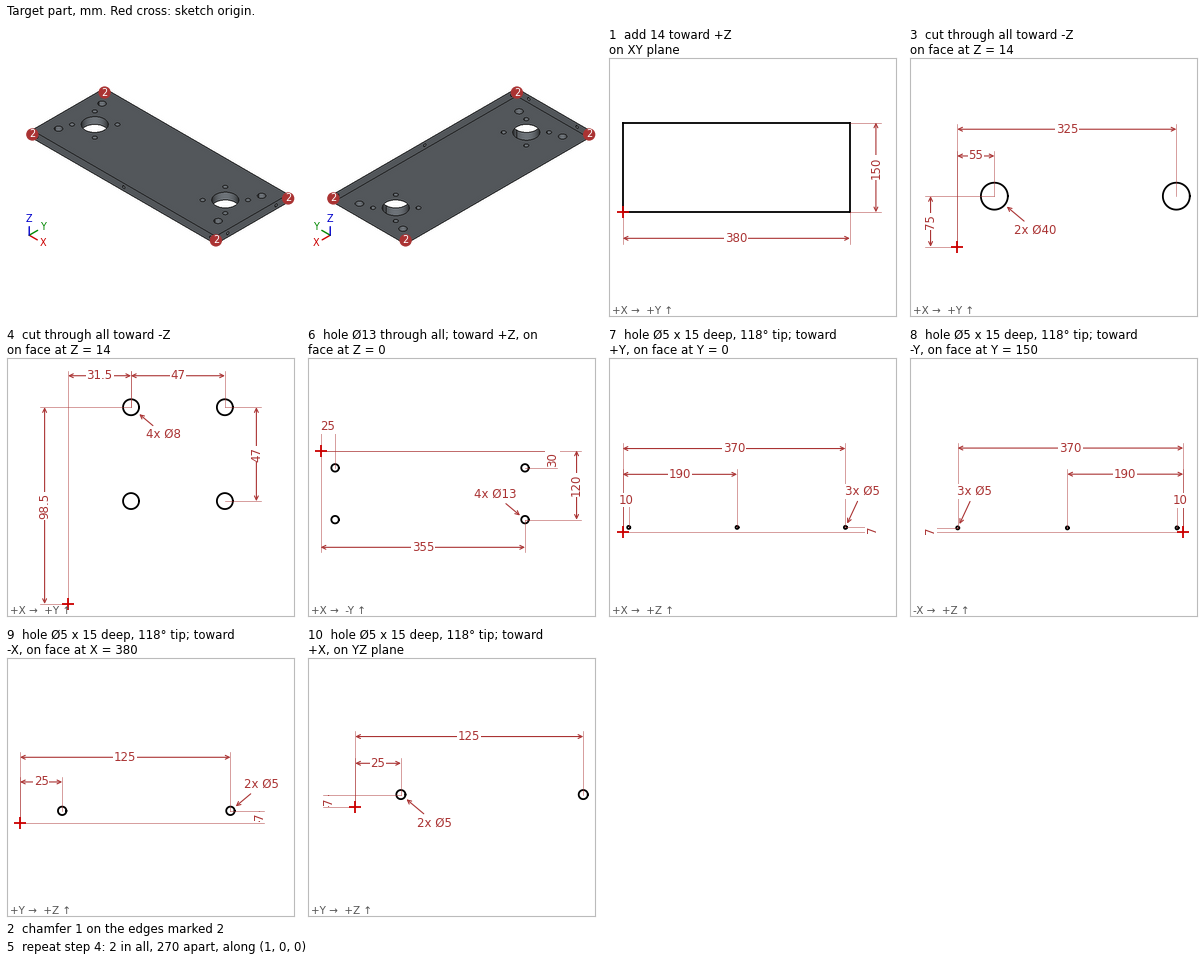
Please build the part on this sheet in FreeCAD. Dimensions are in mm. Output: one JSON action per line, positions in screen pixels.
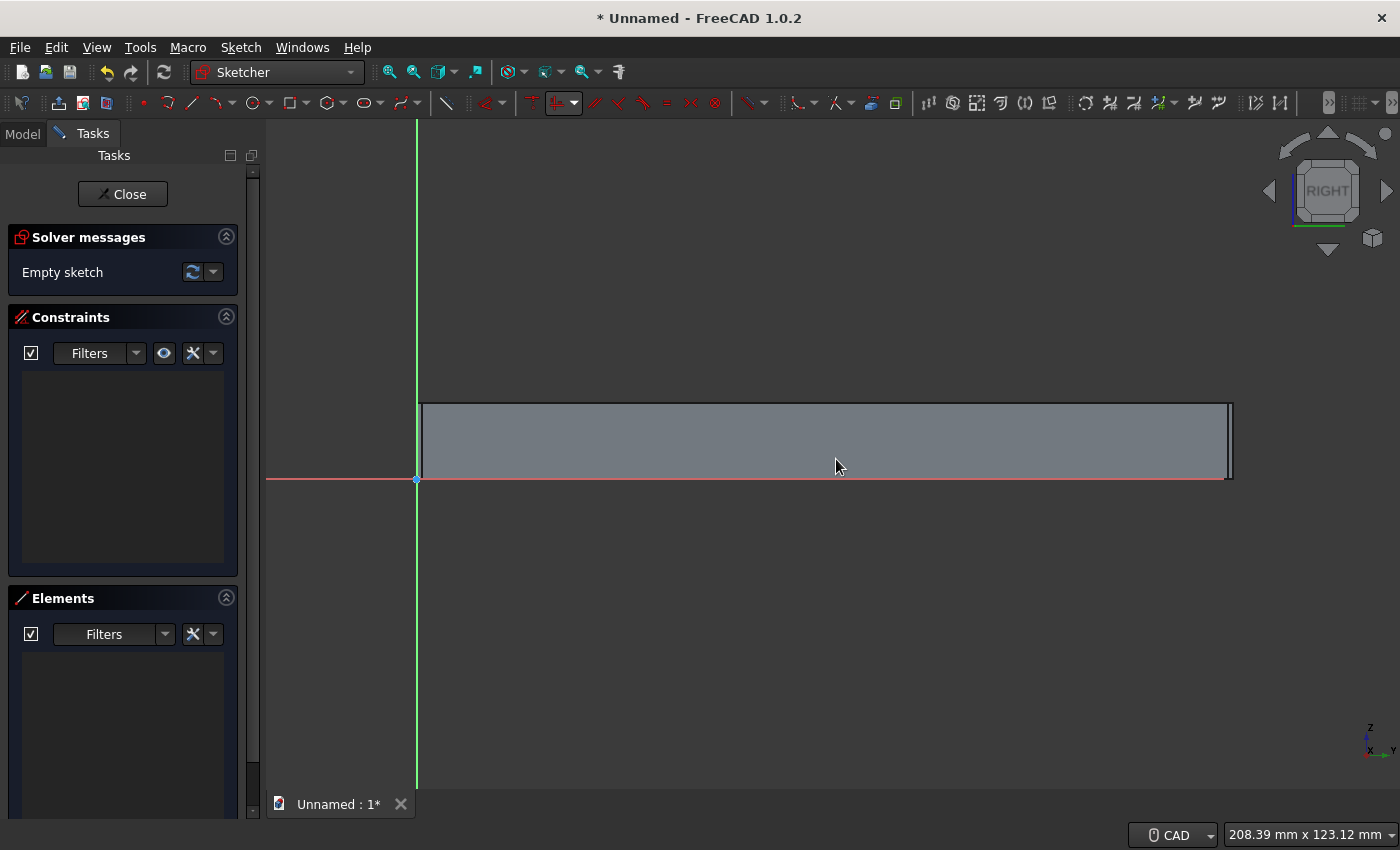
{"action": "key", "text": "g c"}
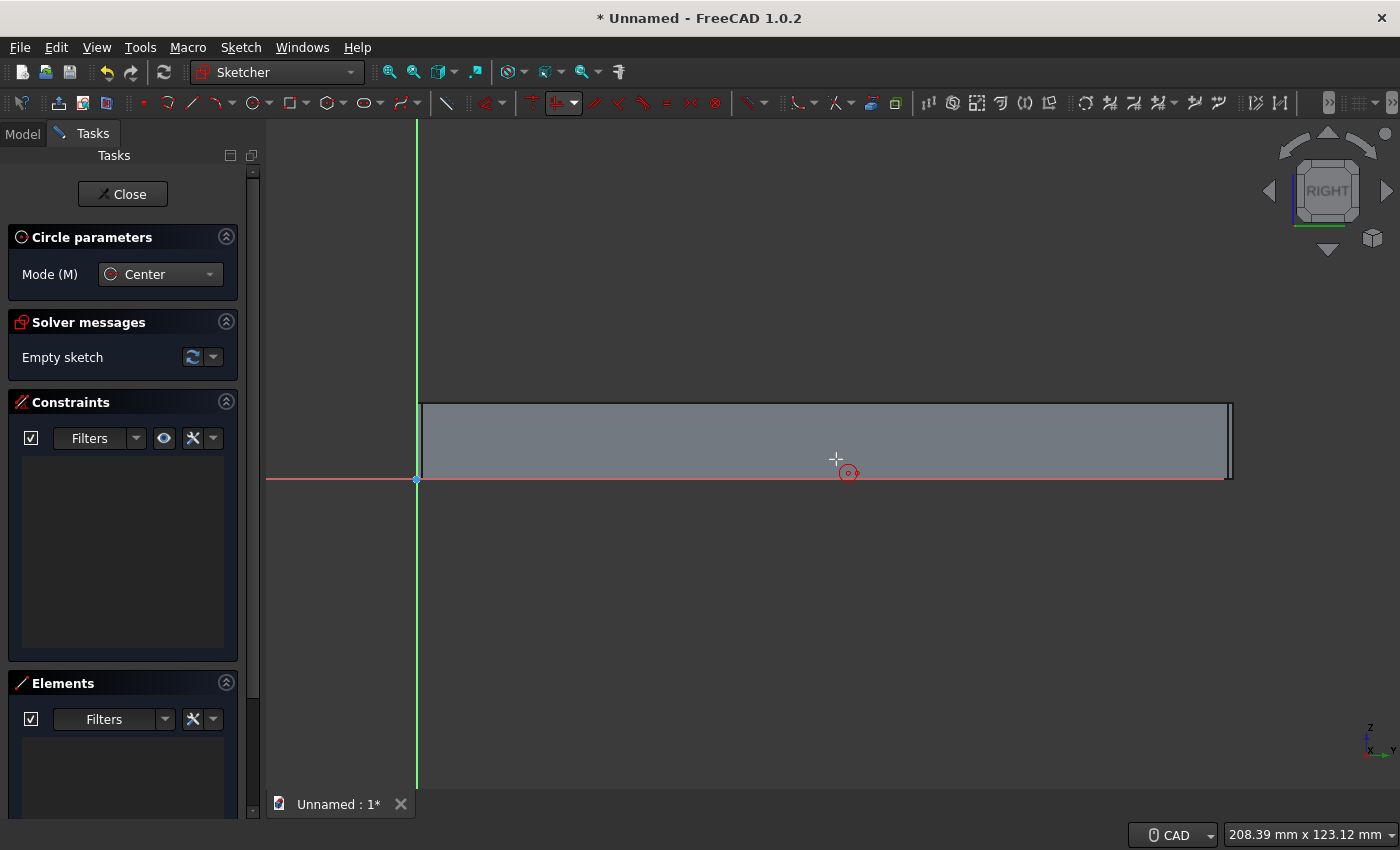
{"action": "scroll", "coordinate": [1097, 441], "scroll_direction": "up", "scroll_amount": 3}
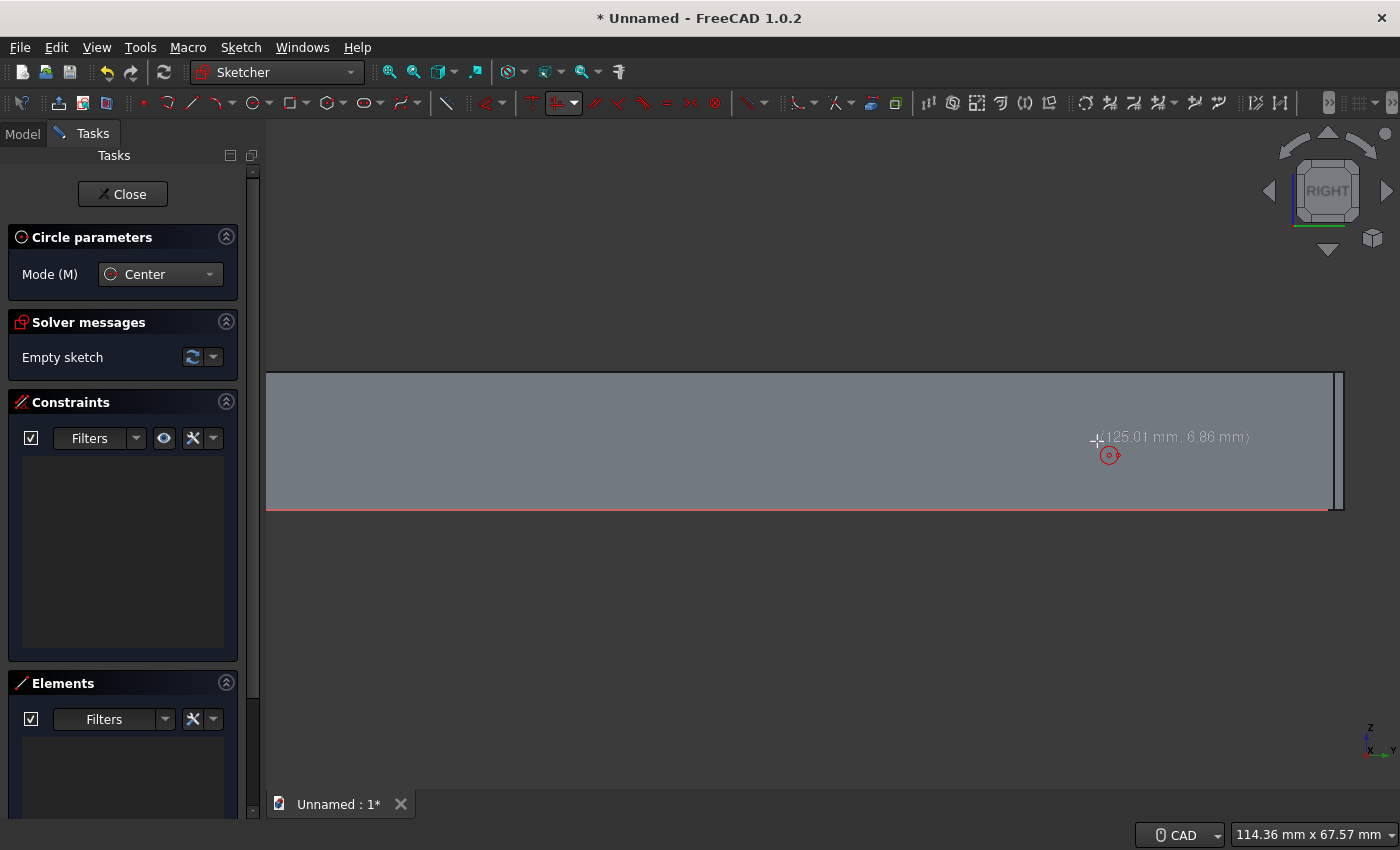
{"action": "left_click", "coordinate": [1096, 441]}
{"action": "mouse_move", "coordinate": [1114, 423]}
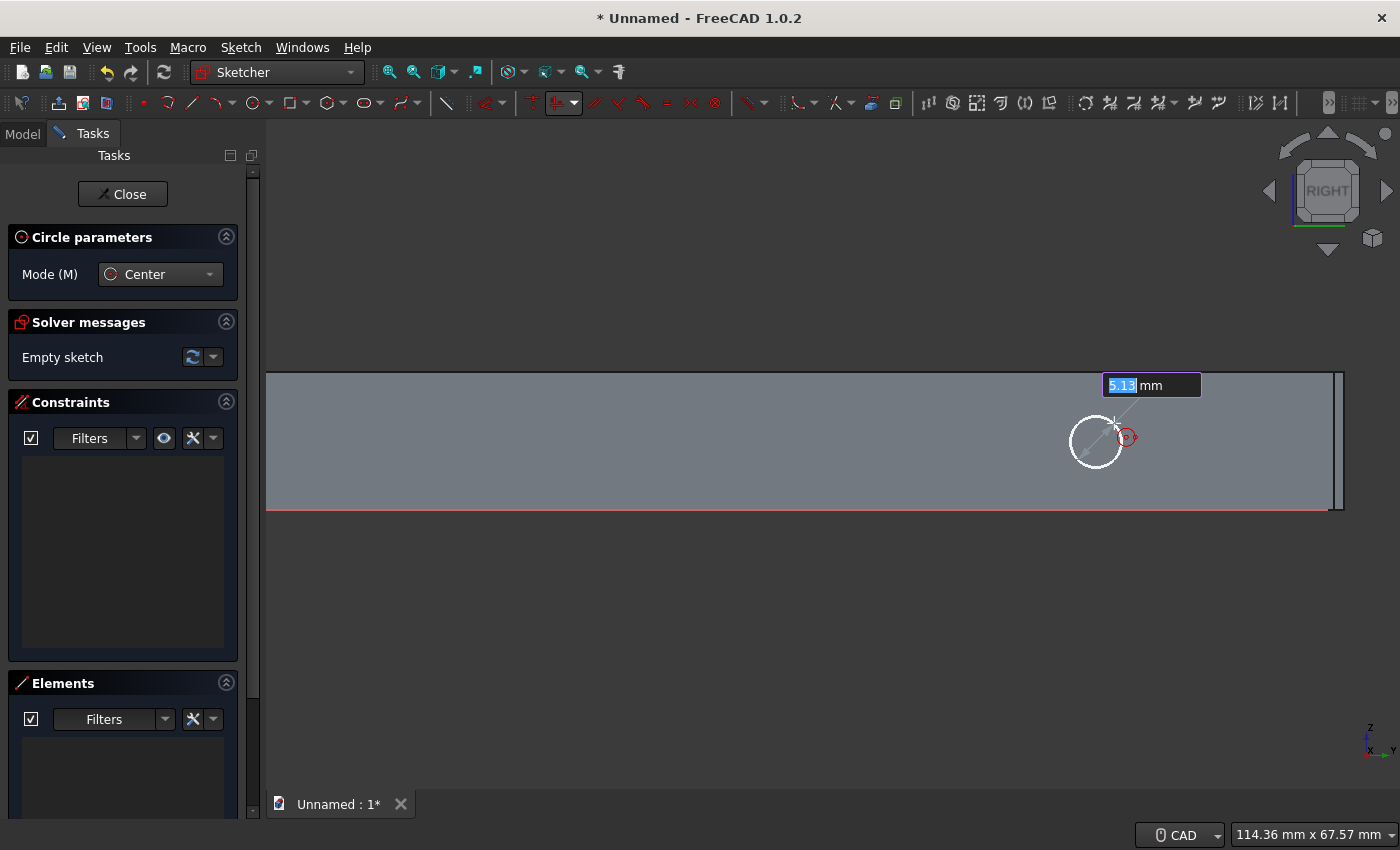
{"action": "type", "text": "5"}
{"action": "key", "text": "Return"}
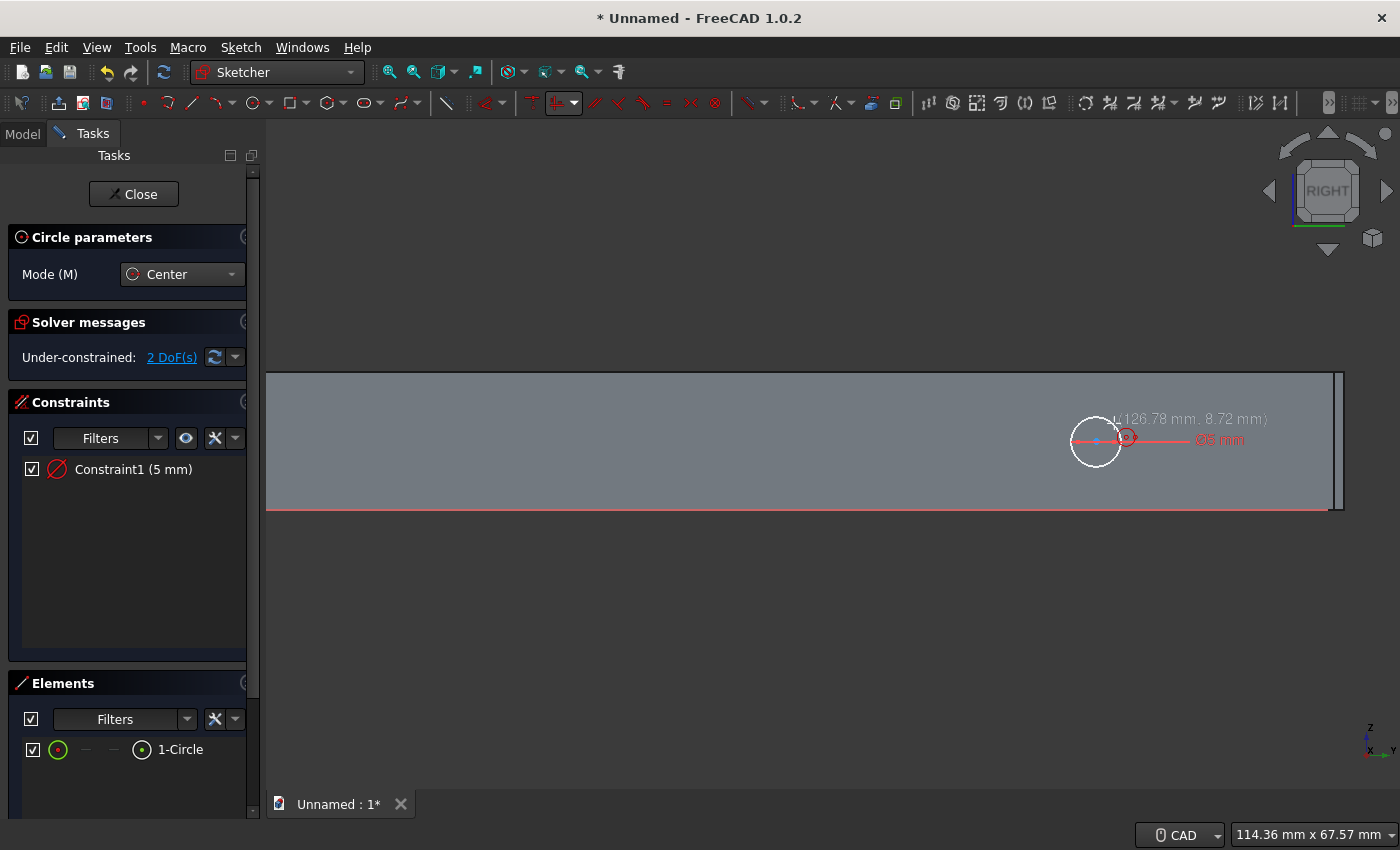
{"action": "scroll", "coordinate": [1100, 443], "scroll_direction": "down", "scroll_amount": 3}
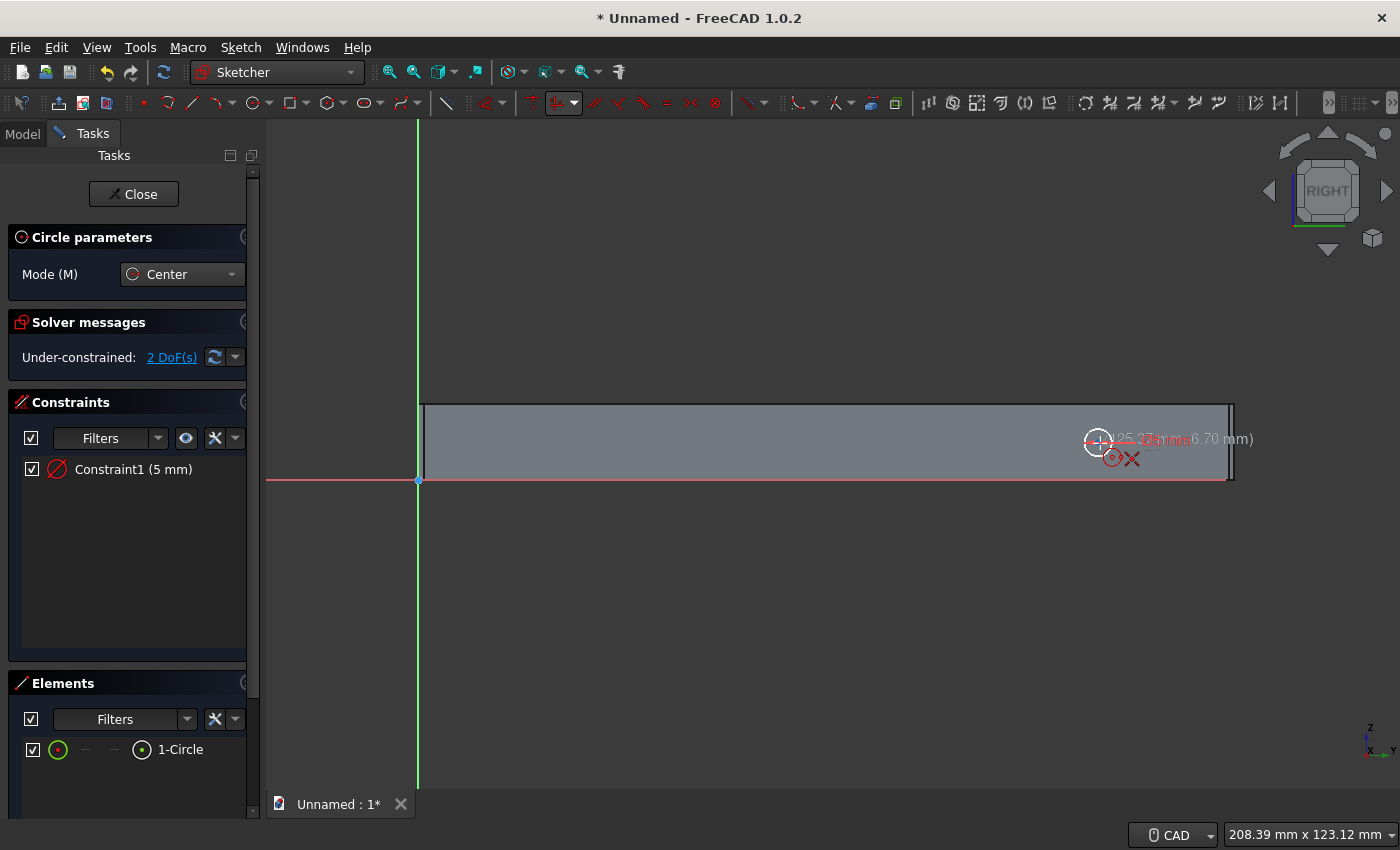
{"action": "scroll", "coordinate": [554, 442], "scroll_direction": "up", "scroll_amount": 3}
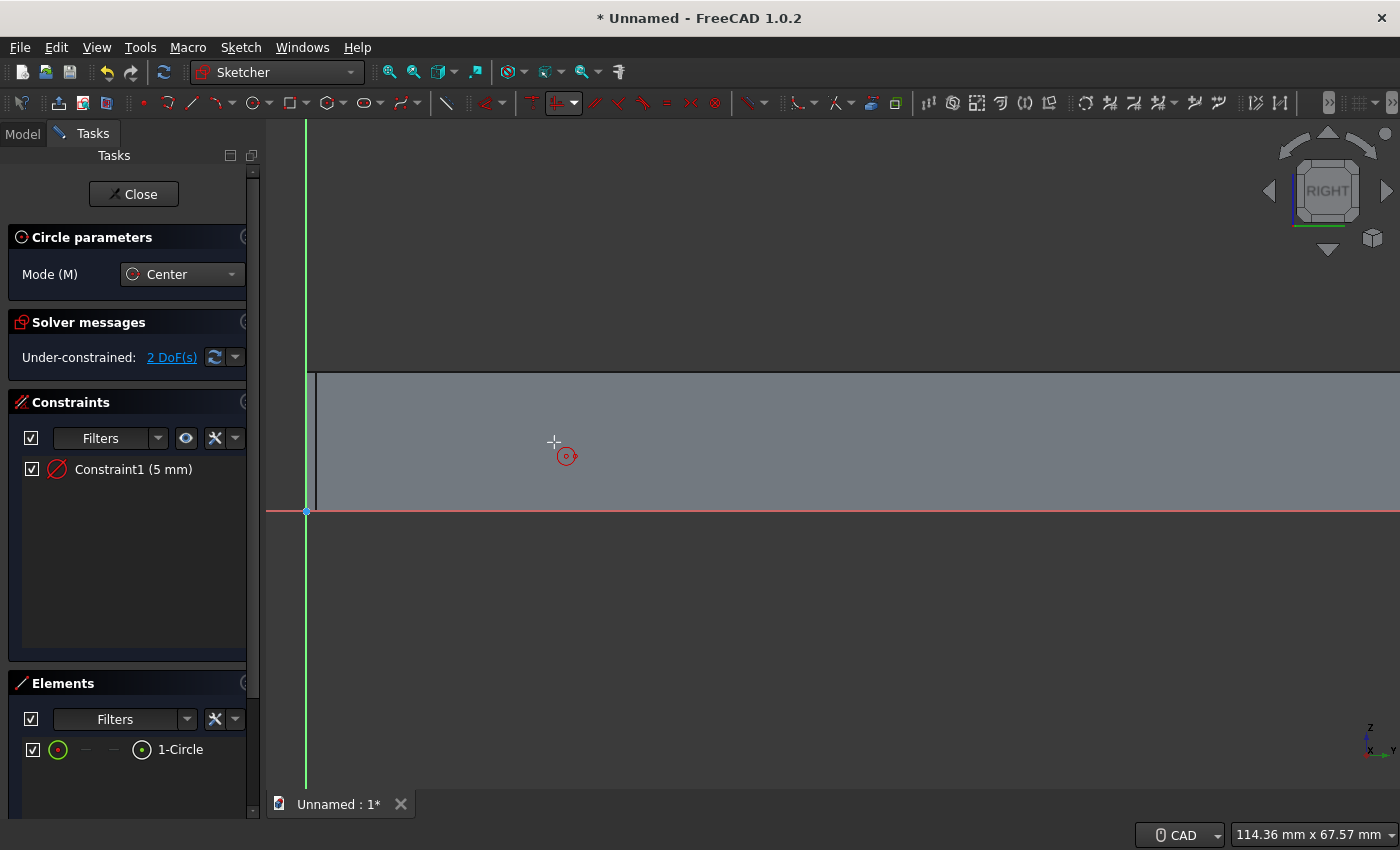
{"action": "left_click", "coordinate": [554, 442]}
{"action": "mouse_move", "coordinate": [572, 424]}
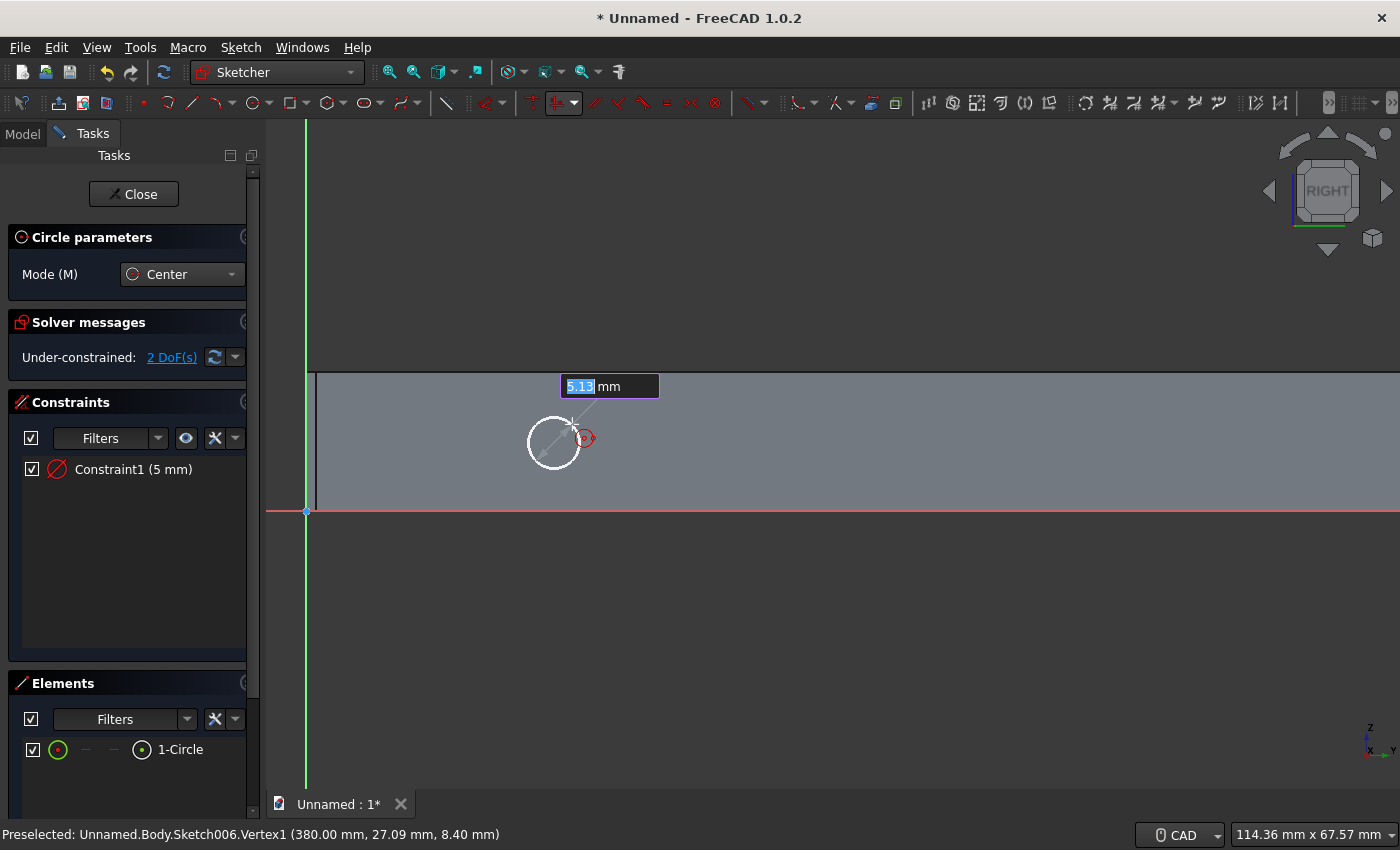
{"action": "type", "text": "5"}
{"action": "key", "text": "Return"}
{"action": "key", "text": "Escape"}